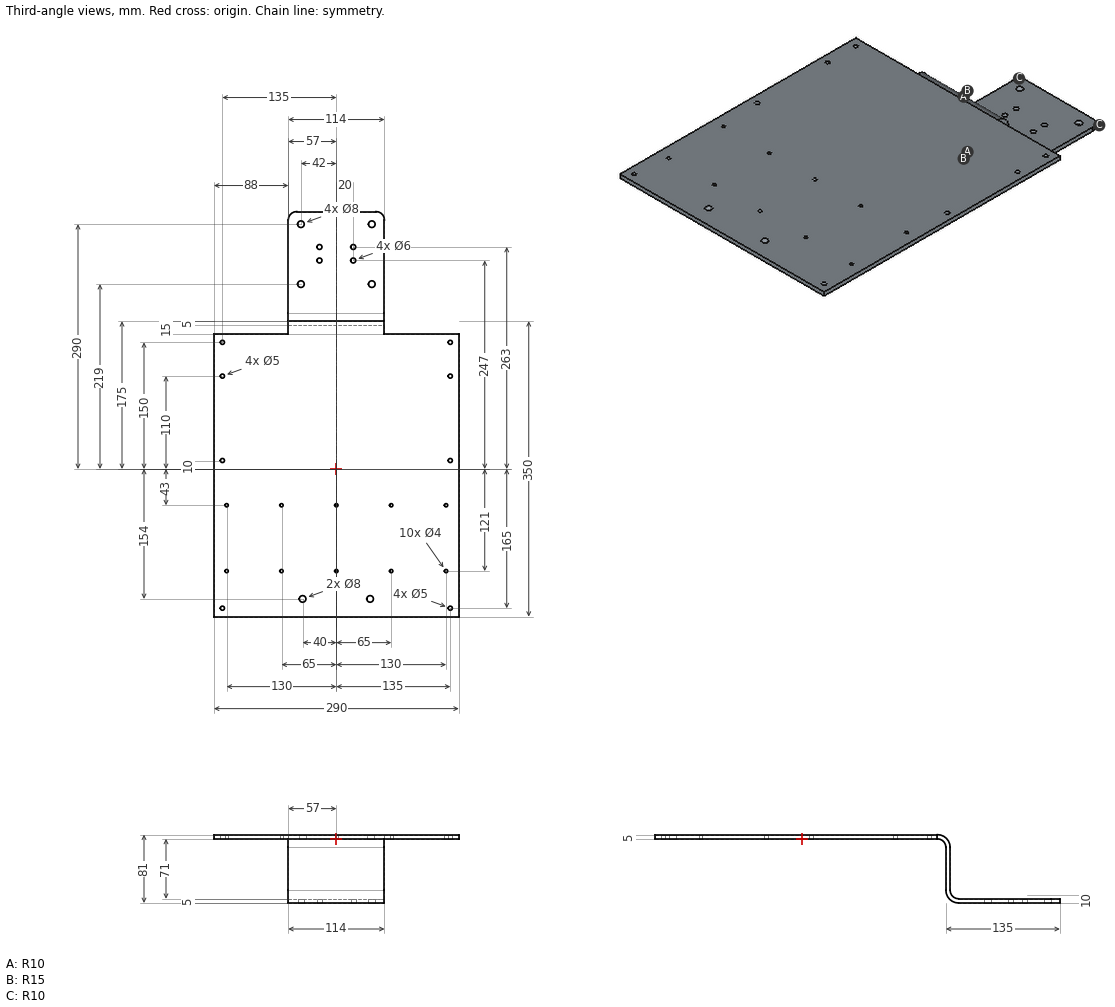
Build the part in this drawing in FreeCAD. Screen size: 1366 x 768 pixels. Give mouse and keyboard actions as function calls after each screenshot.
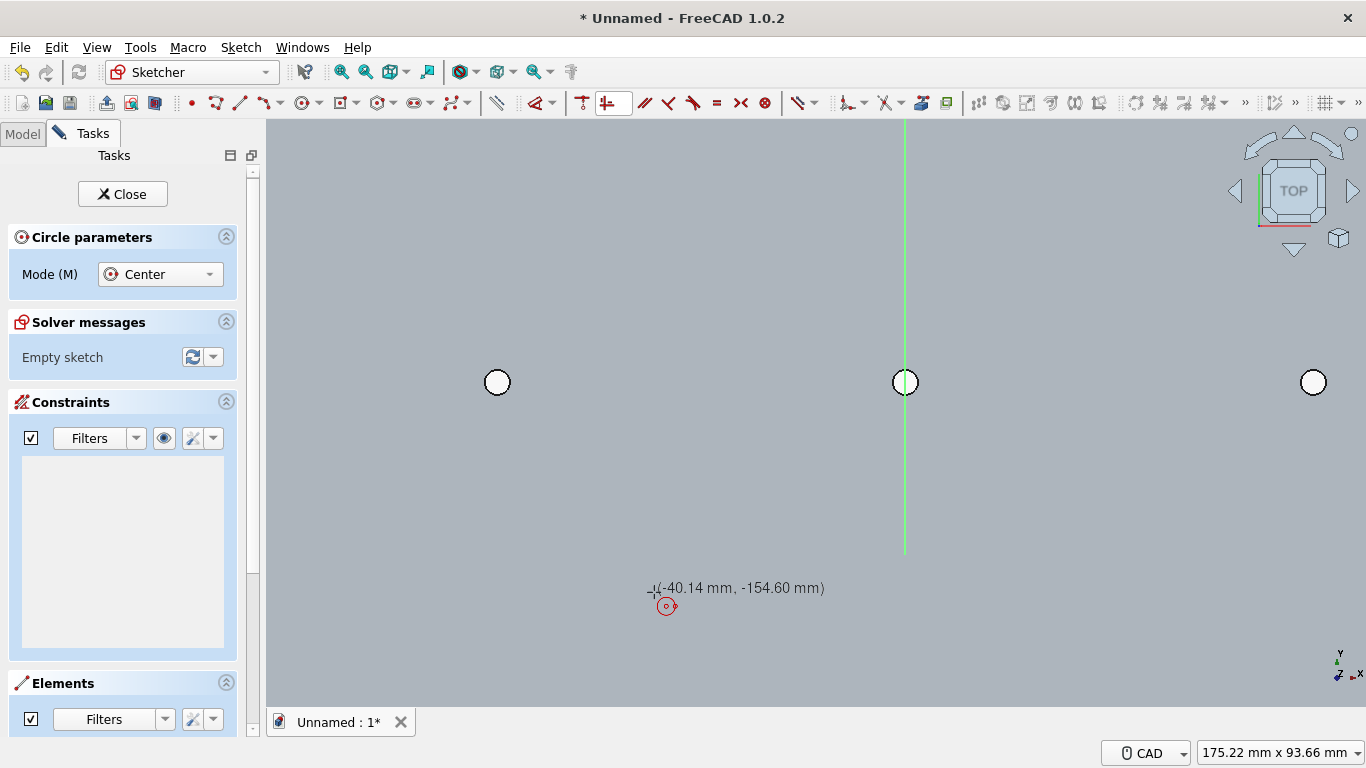
click(654, 590)
click(672, 572)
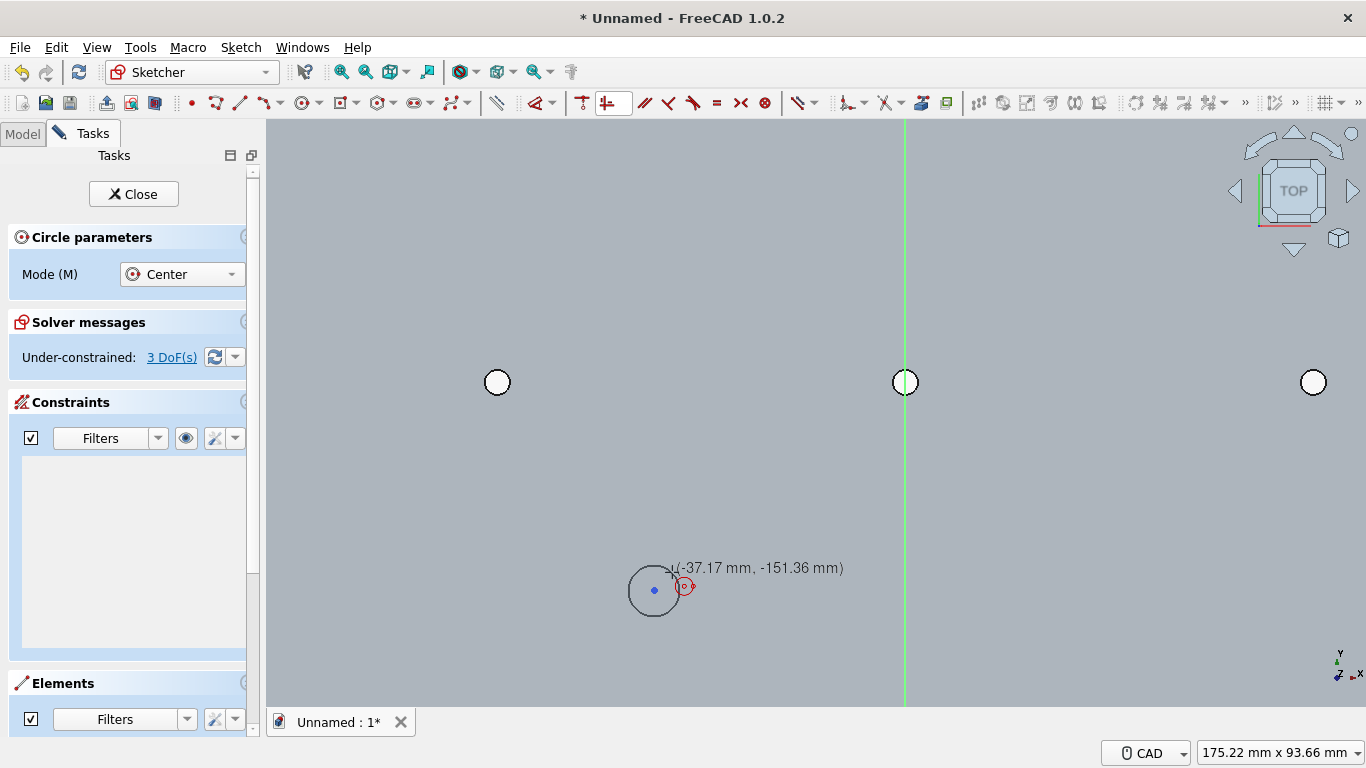
click(1156, 590)
click(1174, 572)
key(Escape)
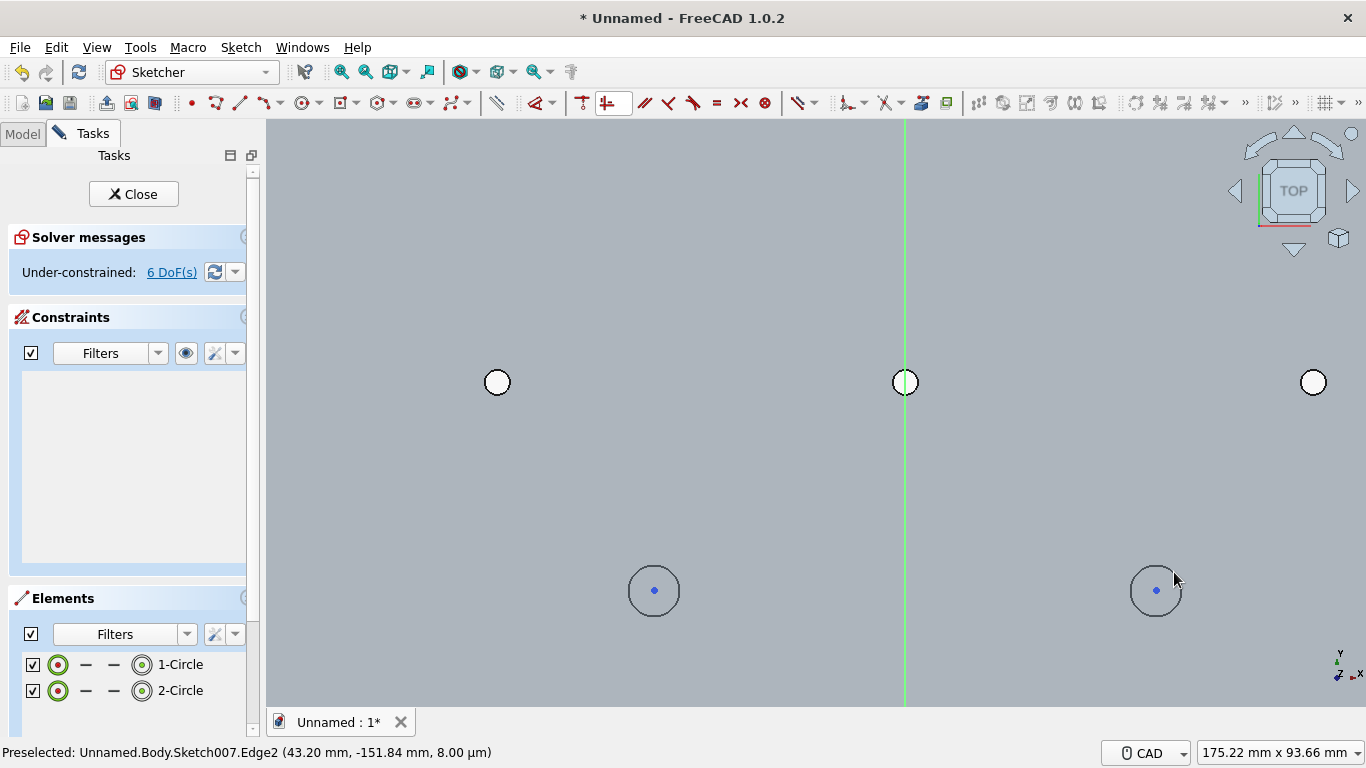
click(672, 573)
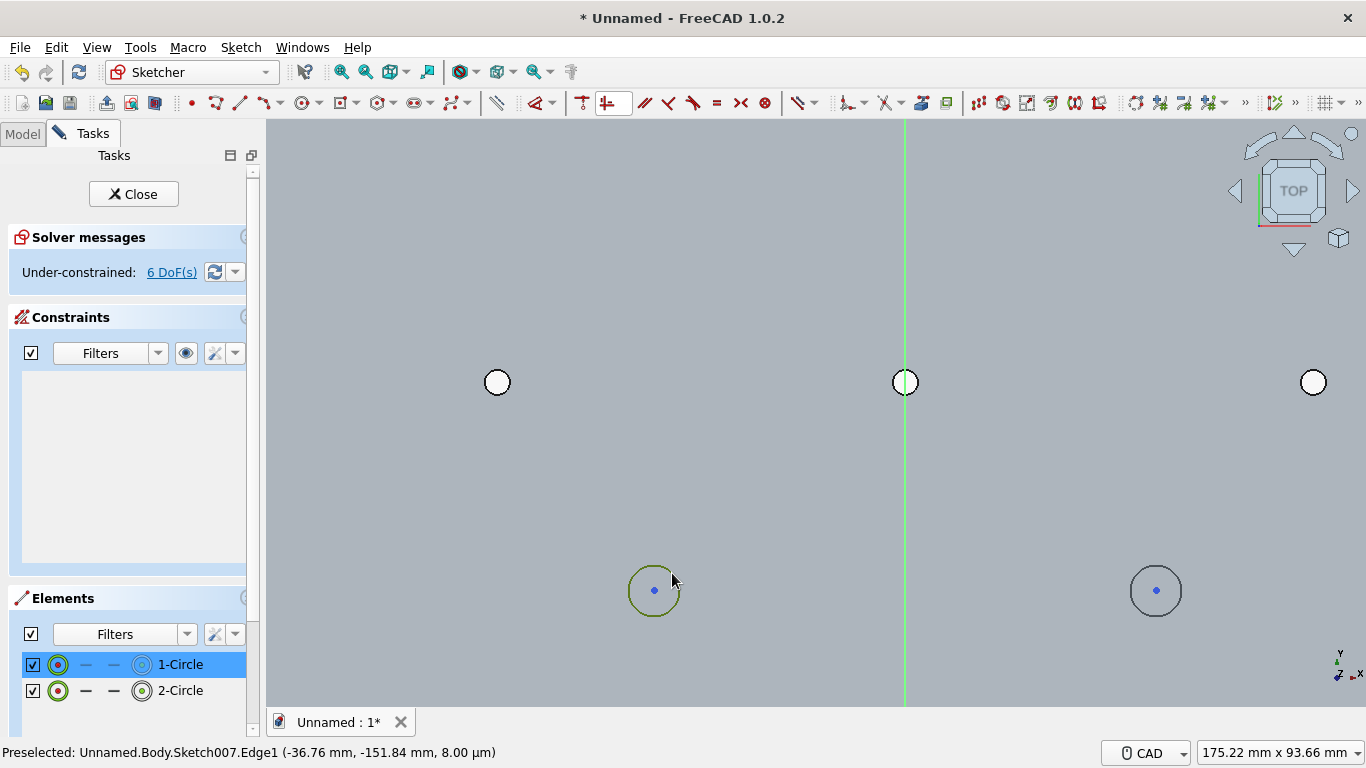
click(1174, 573)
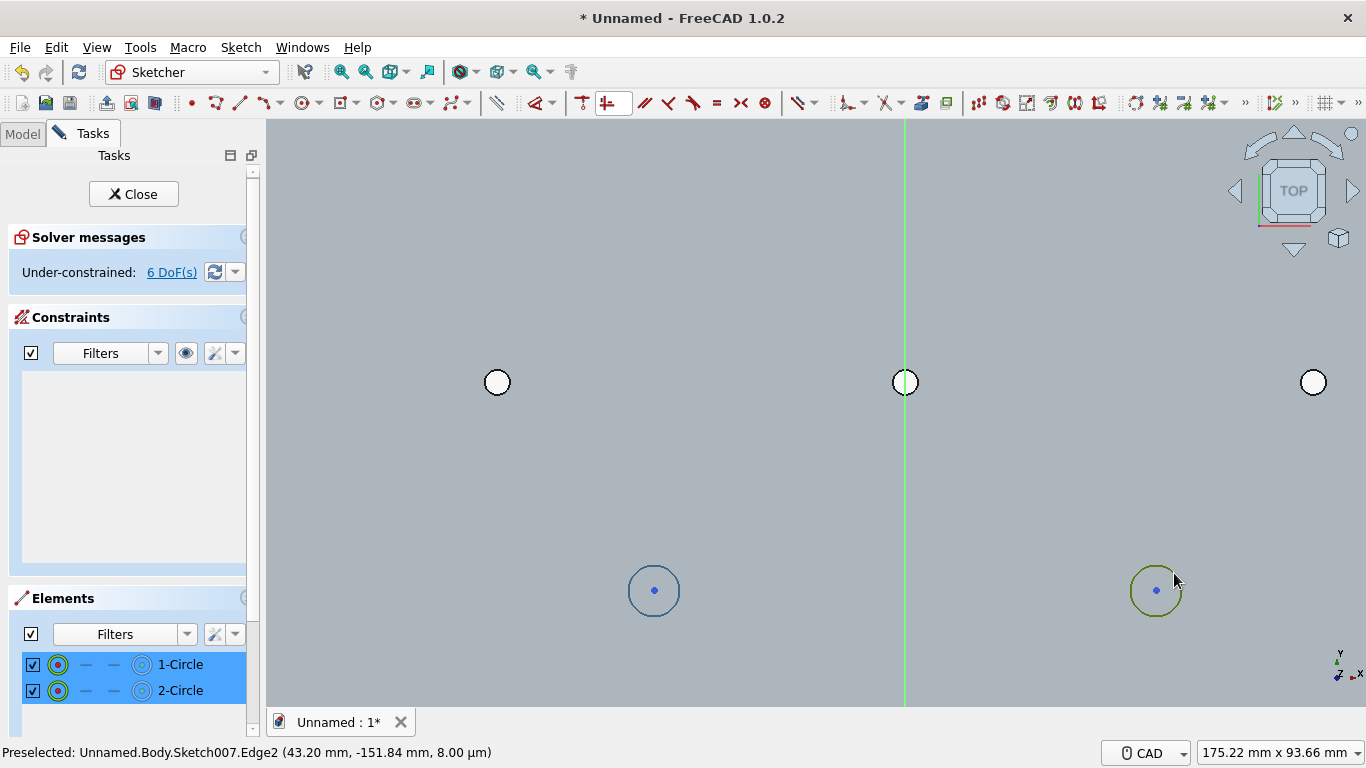
click(718, 104)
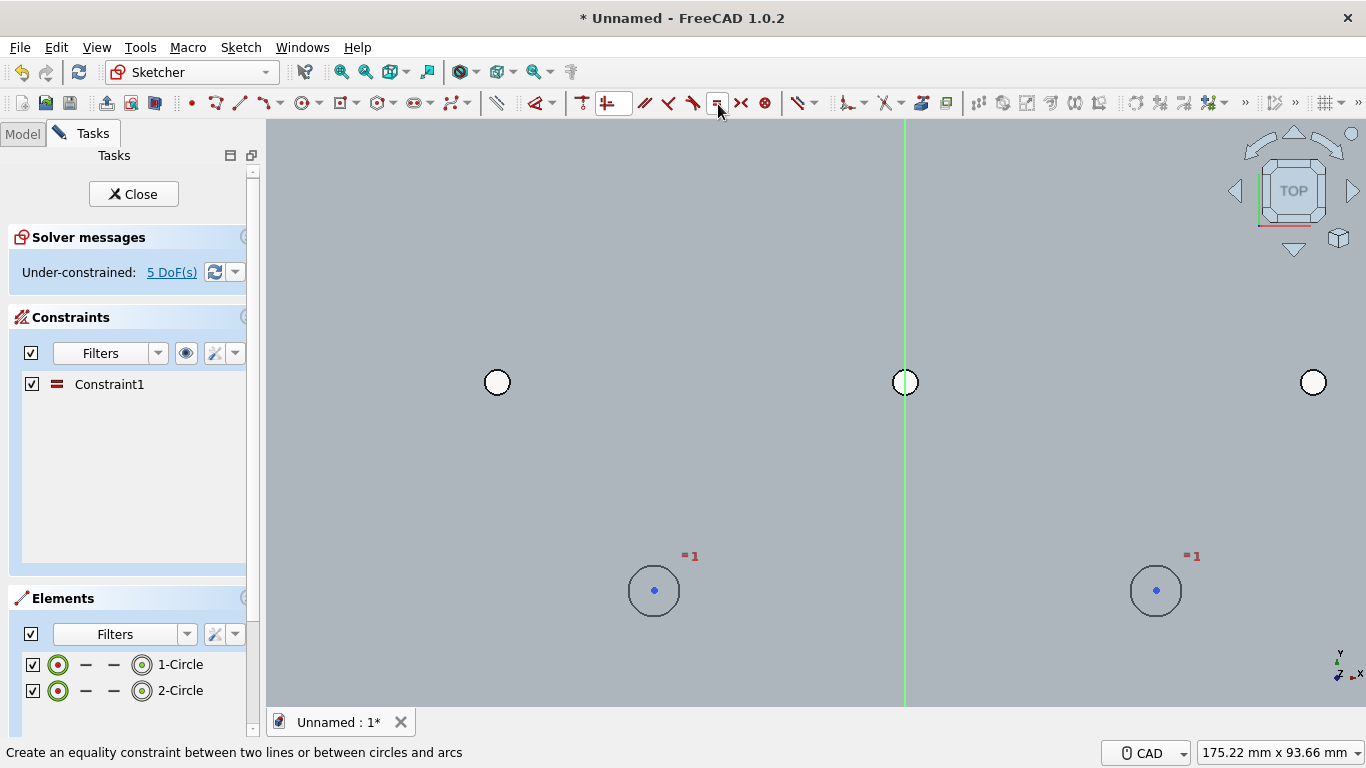
click(654, 591)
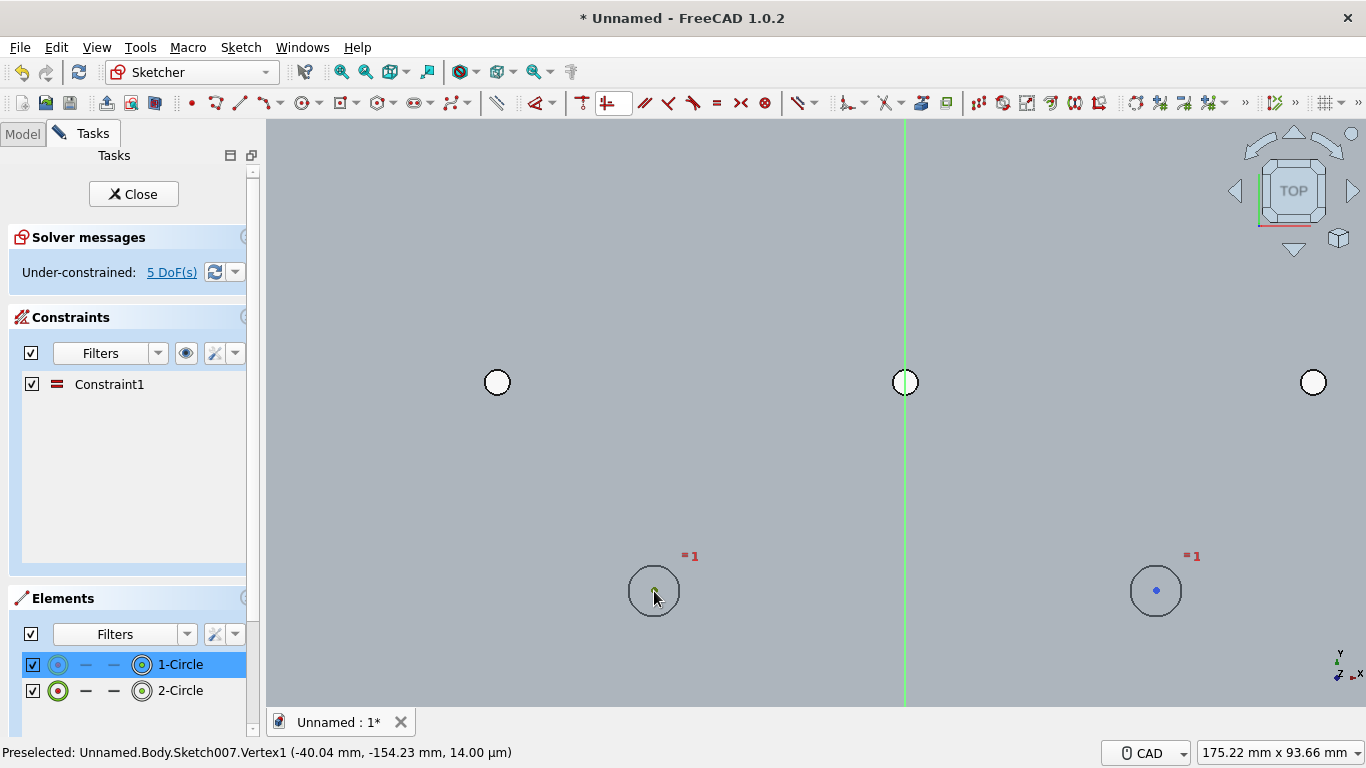
click(1156, 591)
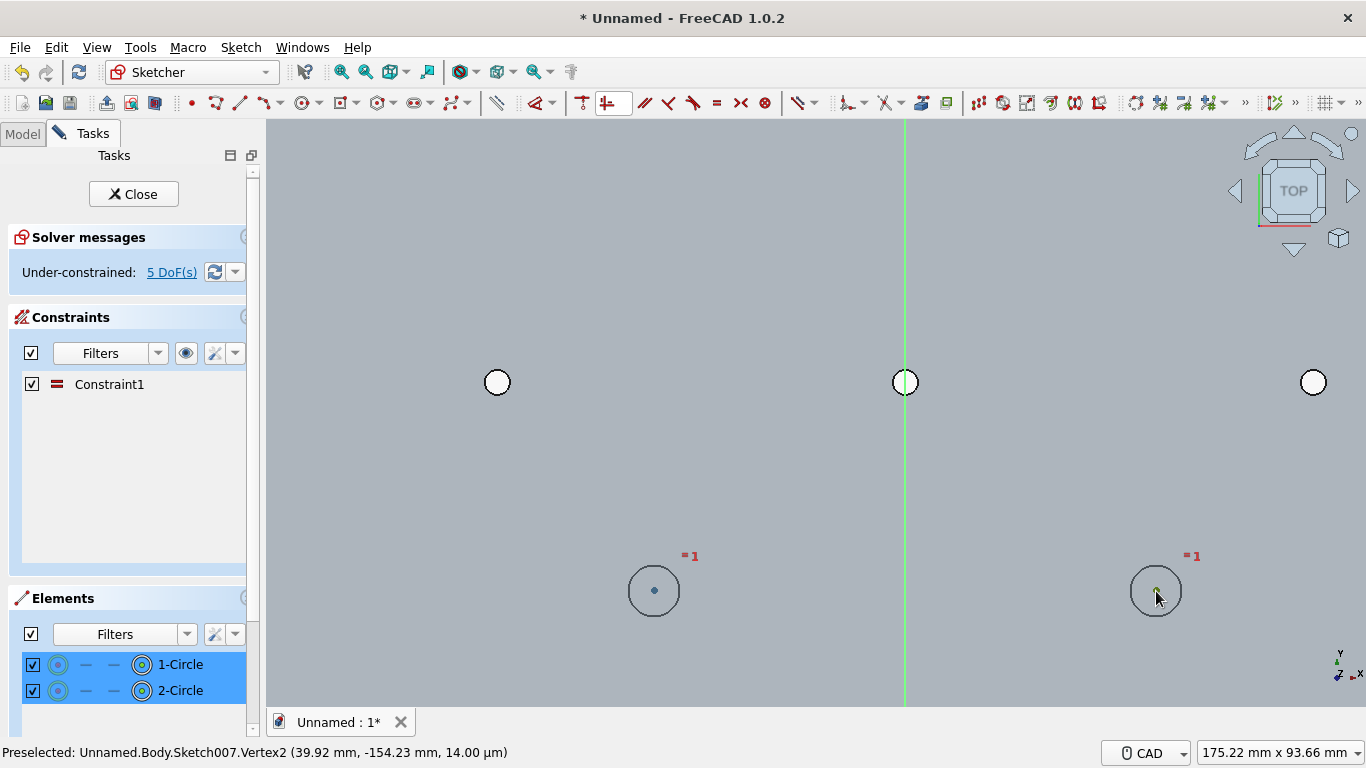
click(905, 641)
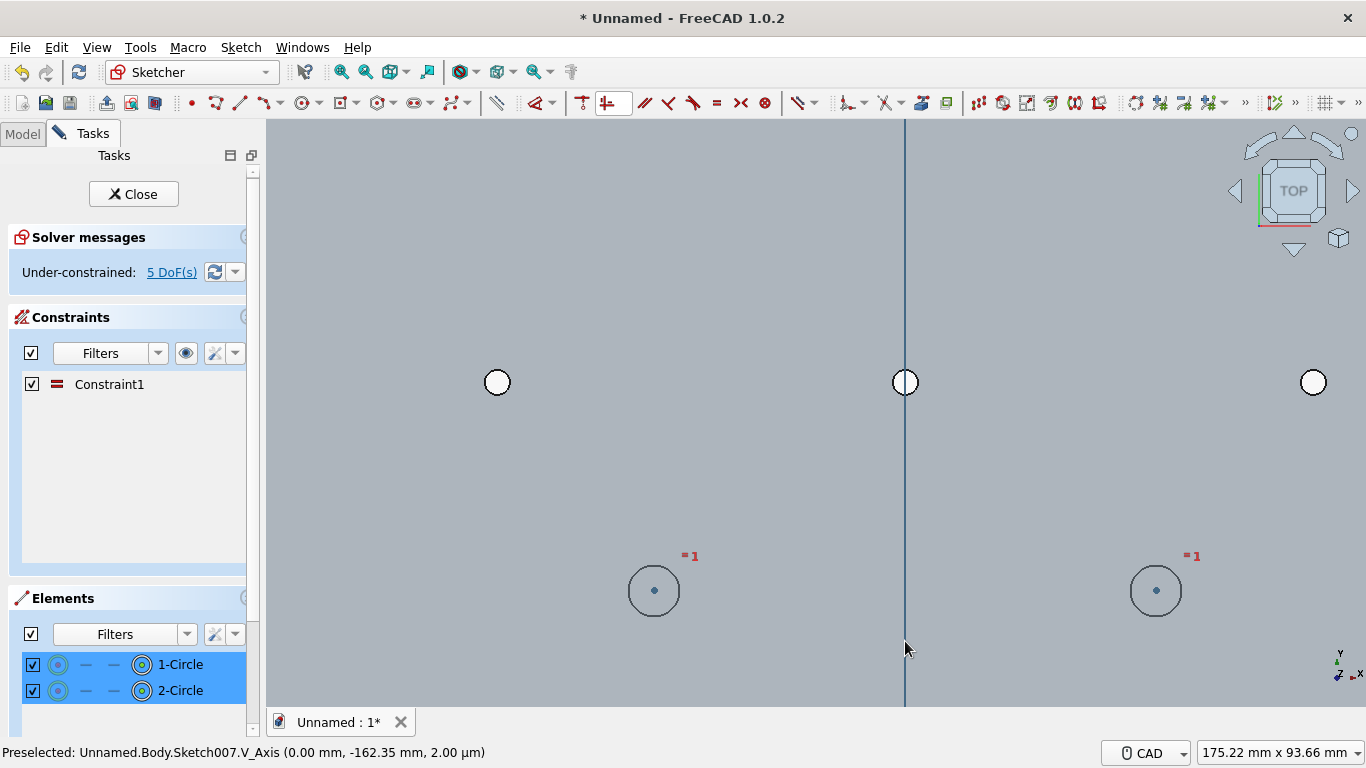
click(742, 104)